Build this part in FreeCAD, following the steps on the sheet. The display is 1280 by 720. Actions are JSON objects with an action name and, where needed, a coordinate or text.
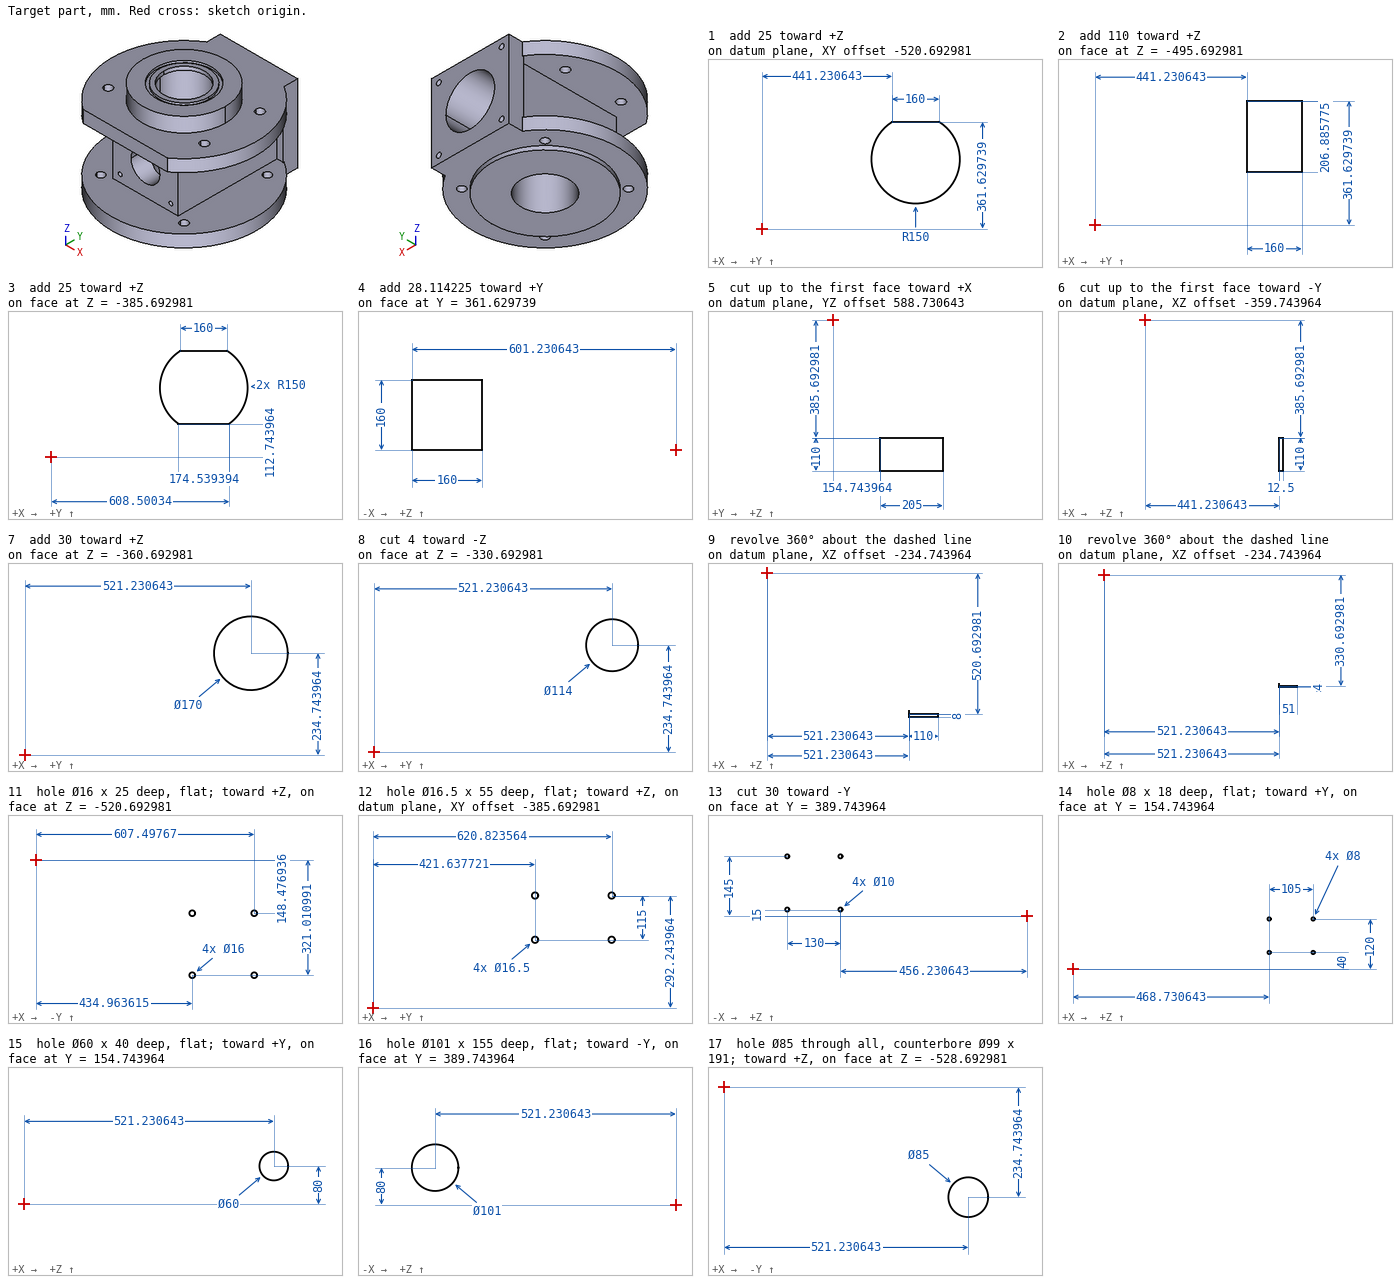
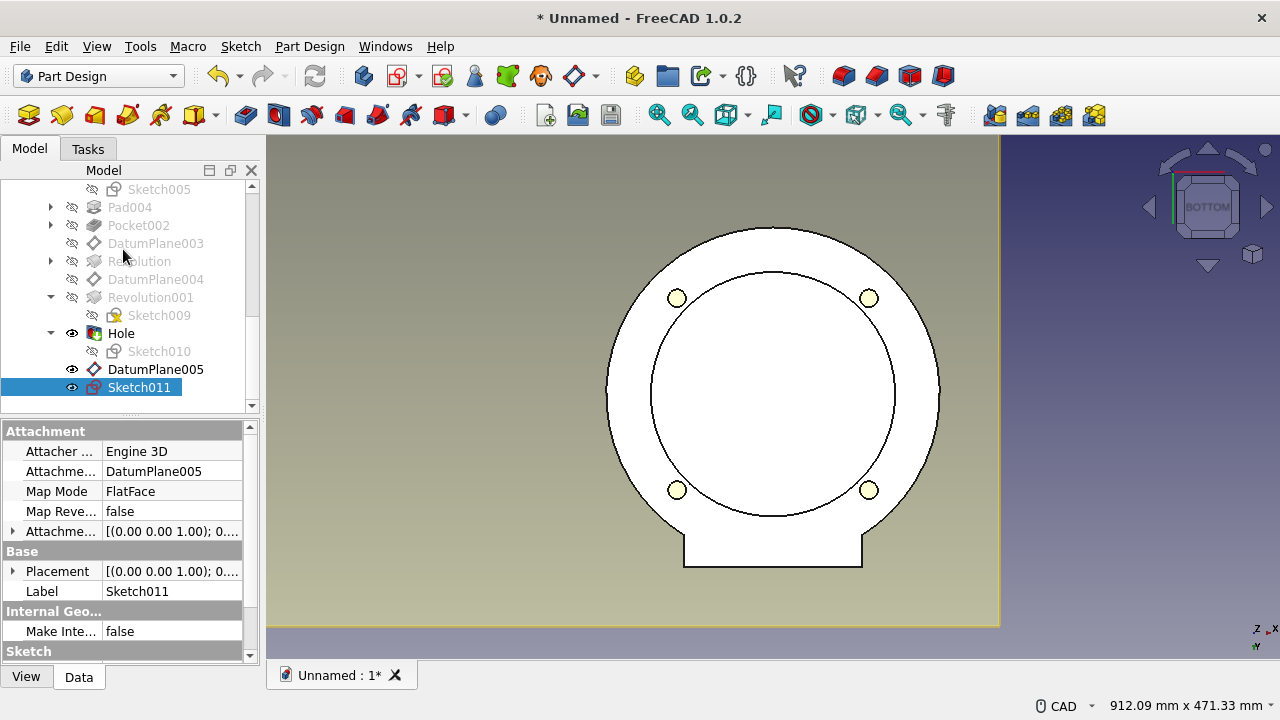
{"action": "left_click", "coordinate": [279, 116]}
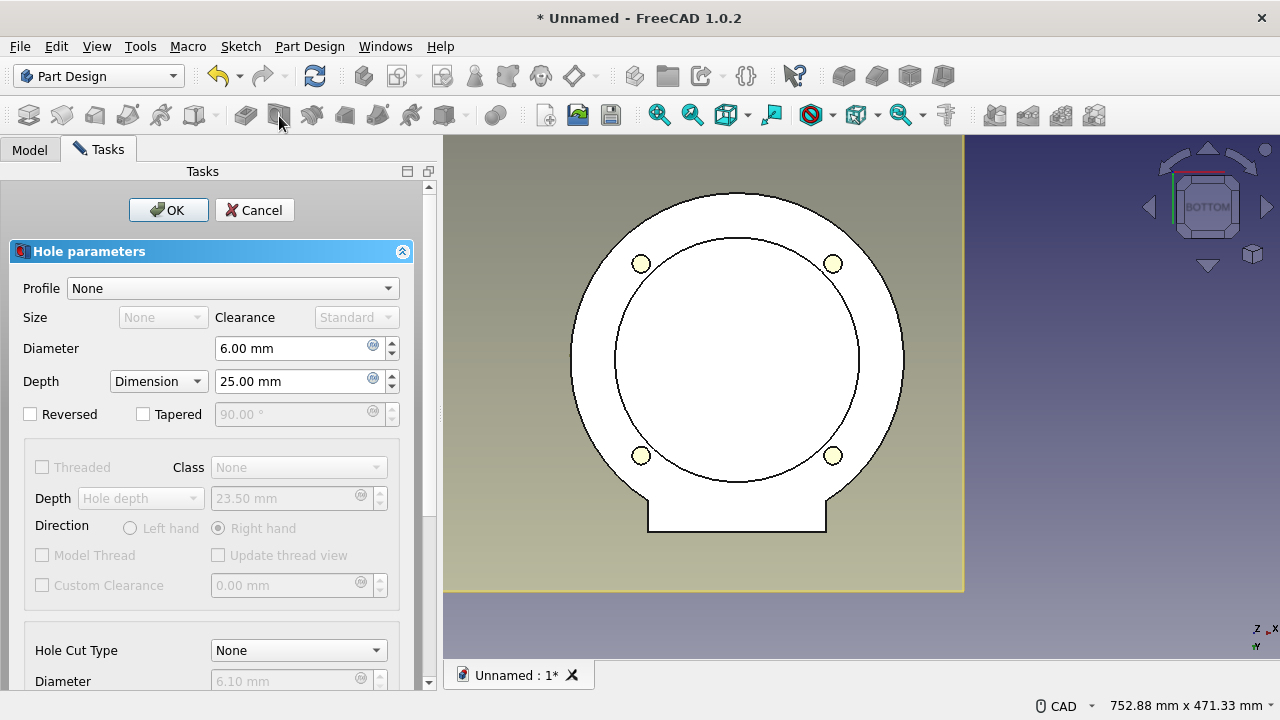
{"action": "triple_click", "coordinate": [300, 348]}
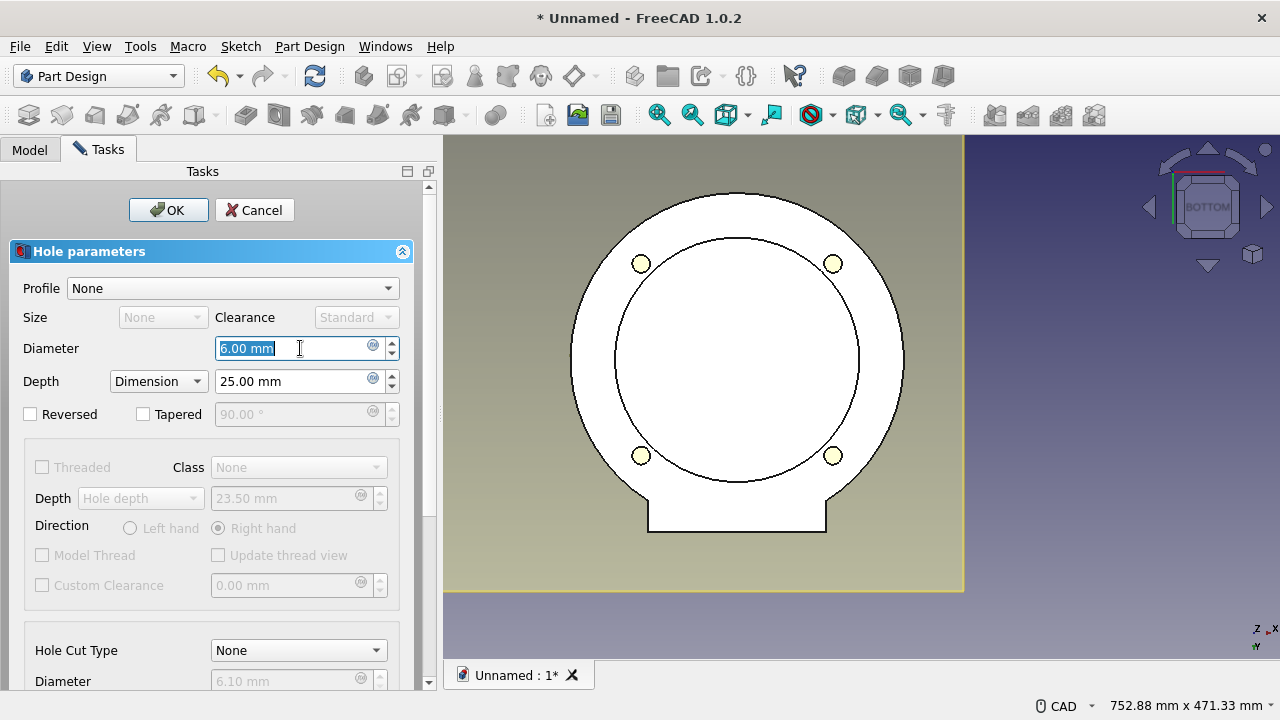
{"action": "type", "text": "16.5"}
{"action": "key", "text": "Tab"}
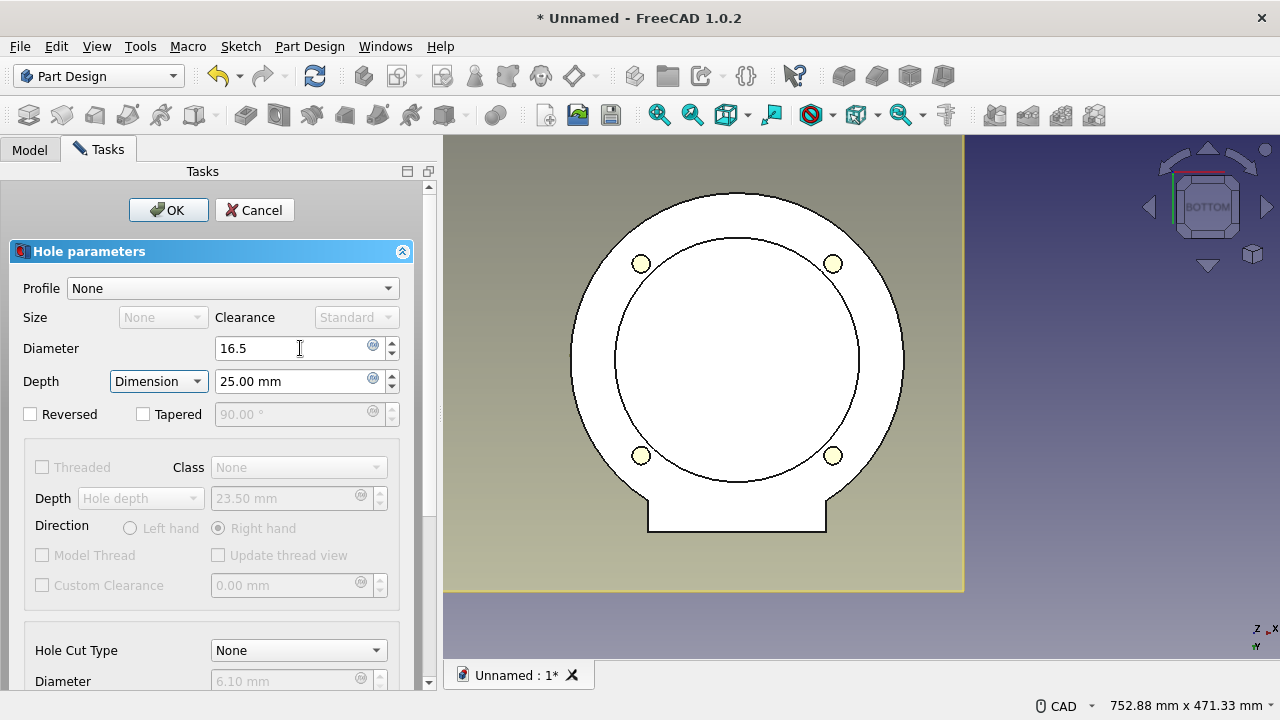
{"action": "triple_click", "coordinate": [300, 382]}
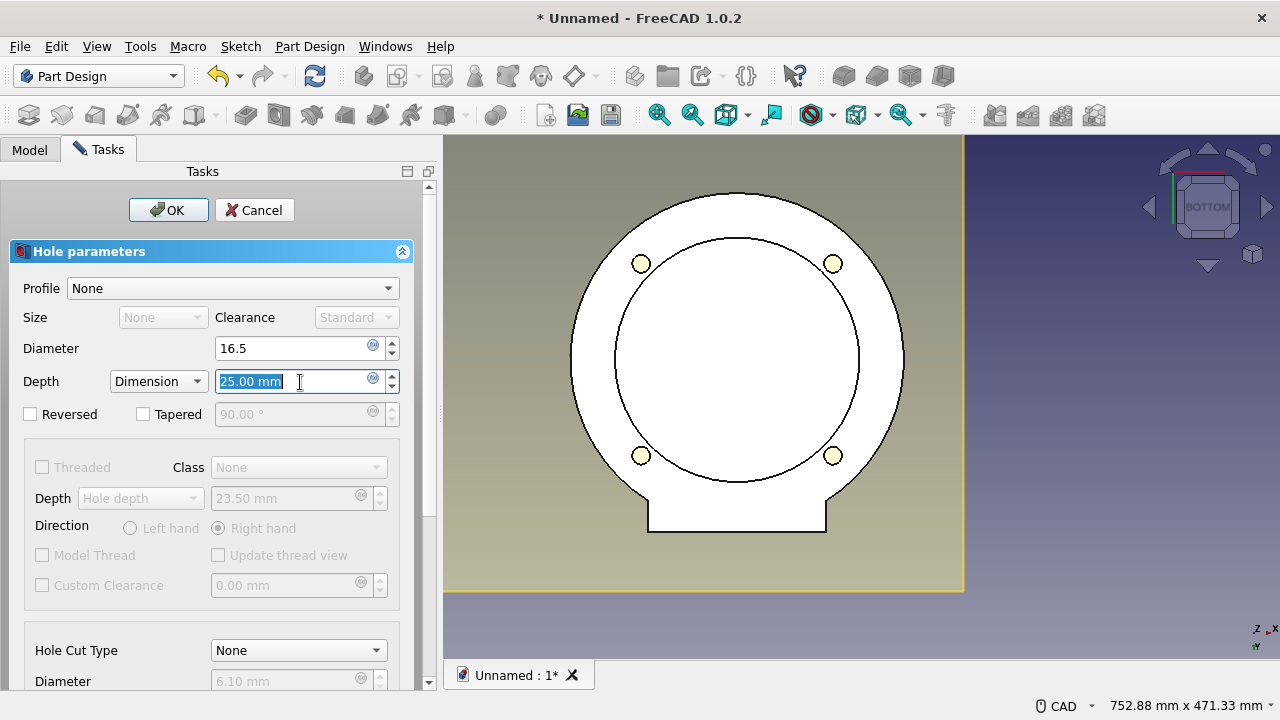
{"action": "type", "text": "55"}
{"action": "key", "text": "Tab"}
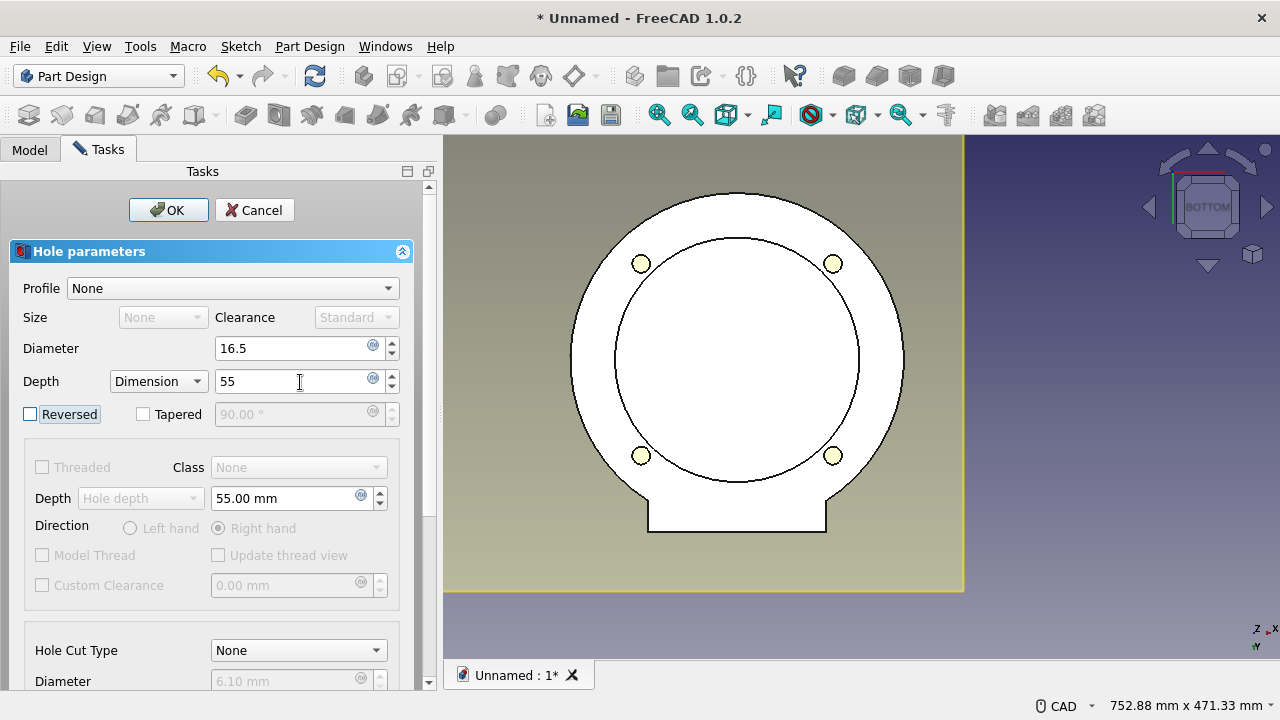
{"action": "left_click", "coordinate": [31, 414]}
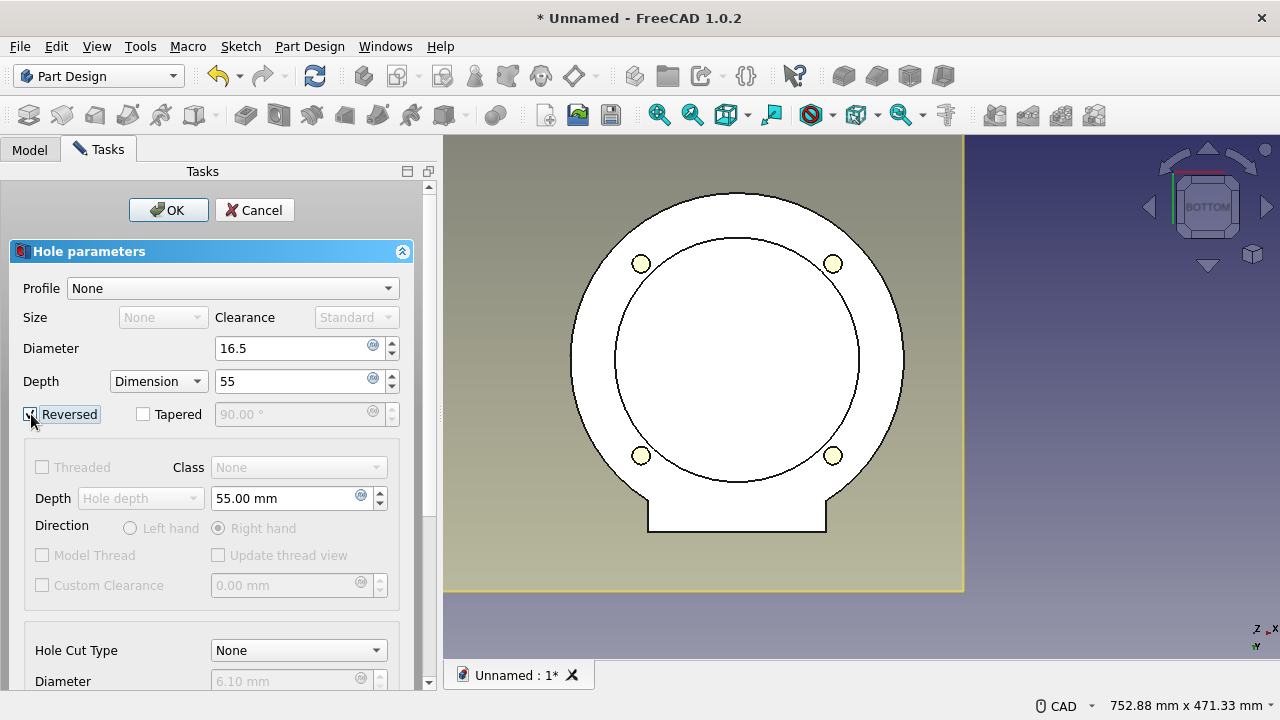
{"action": "scroll", "coordinate": [429, 436], "scroll_direction": "down", "scroll_amount": 4}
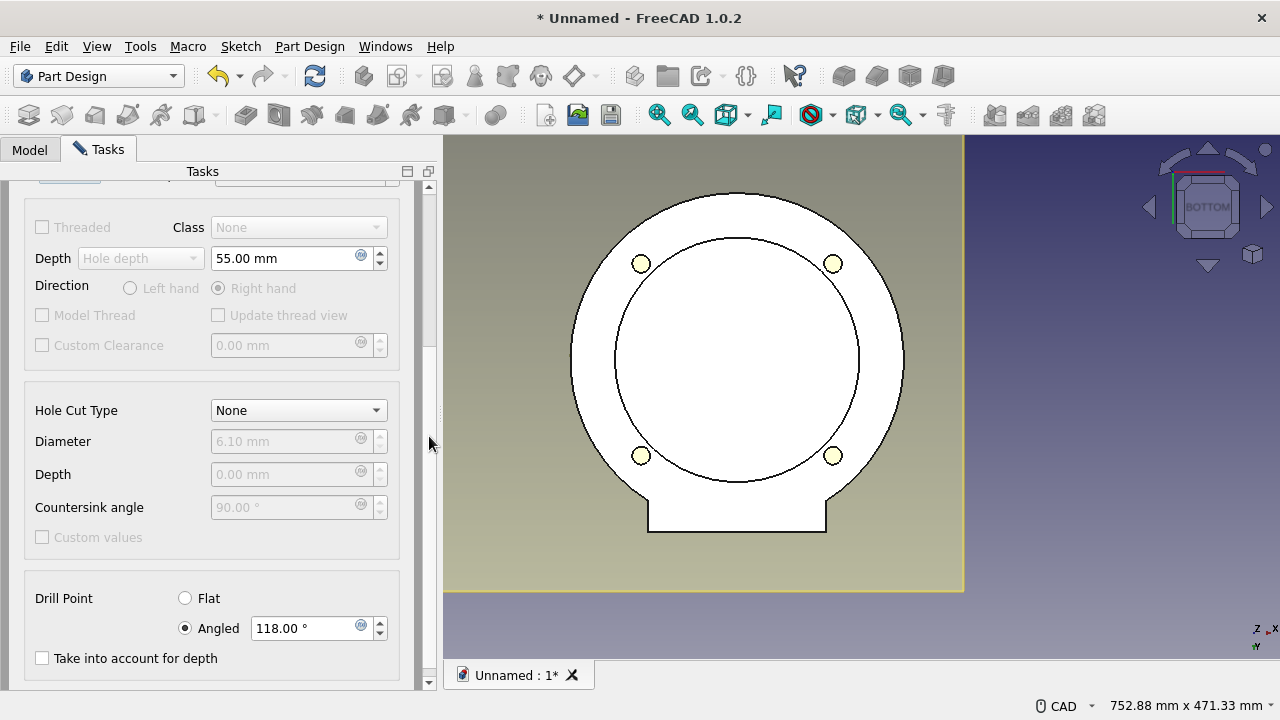
{"action": "left_click", "coordinate": [186, 596]}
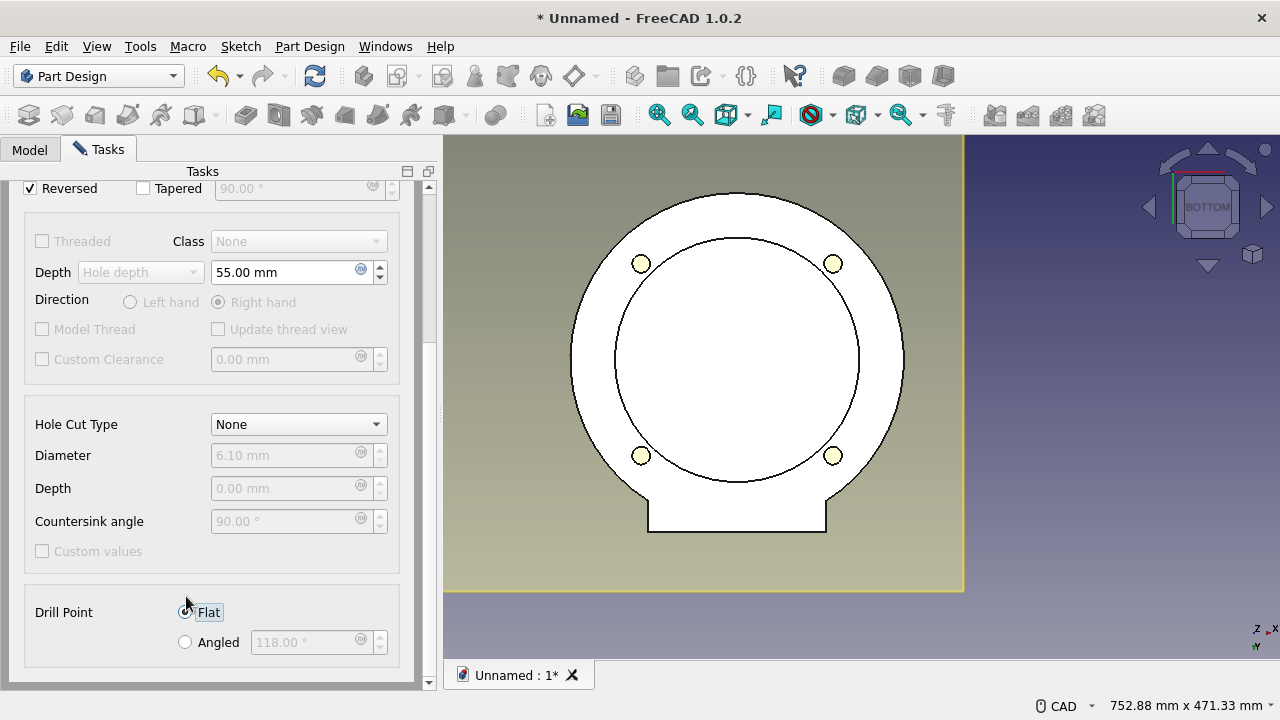
{"action": "scroll", "coordinate": [429, 436], "scroll_direction": "up", "scroll_amount": 5}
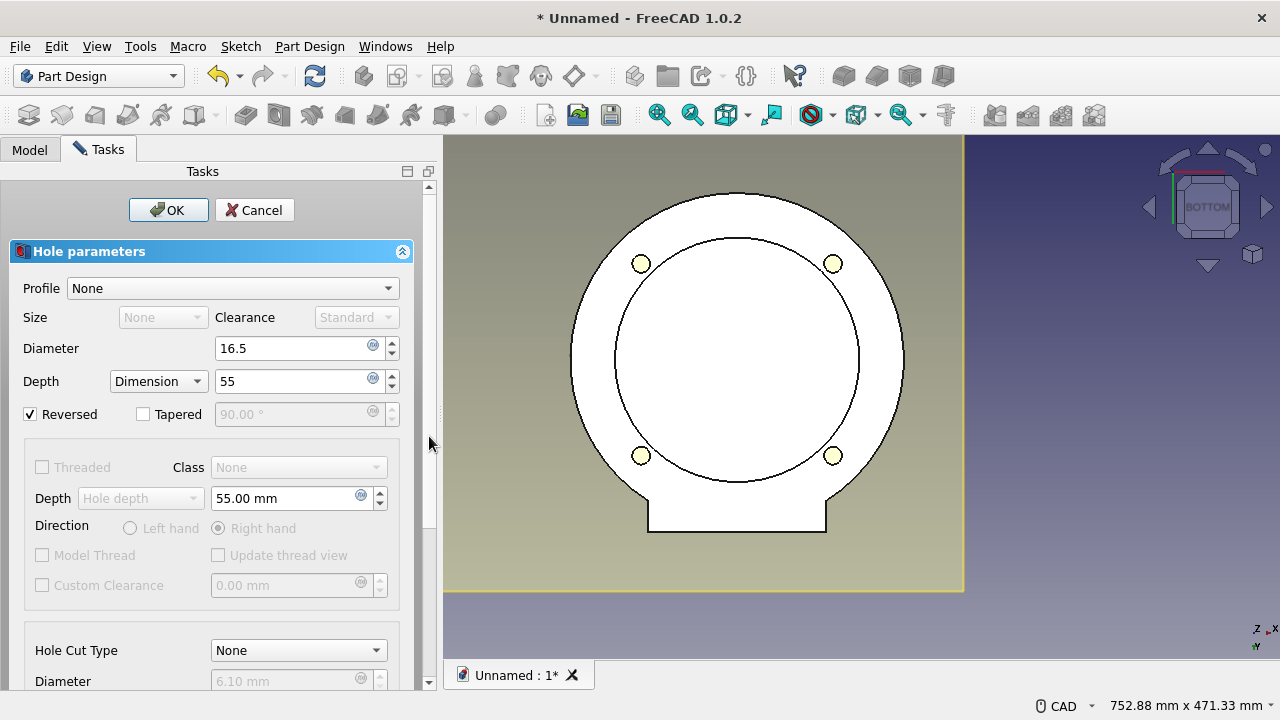
{"action": "left_click", "coordinate": [169, 210]}